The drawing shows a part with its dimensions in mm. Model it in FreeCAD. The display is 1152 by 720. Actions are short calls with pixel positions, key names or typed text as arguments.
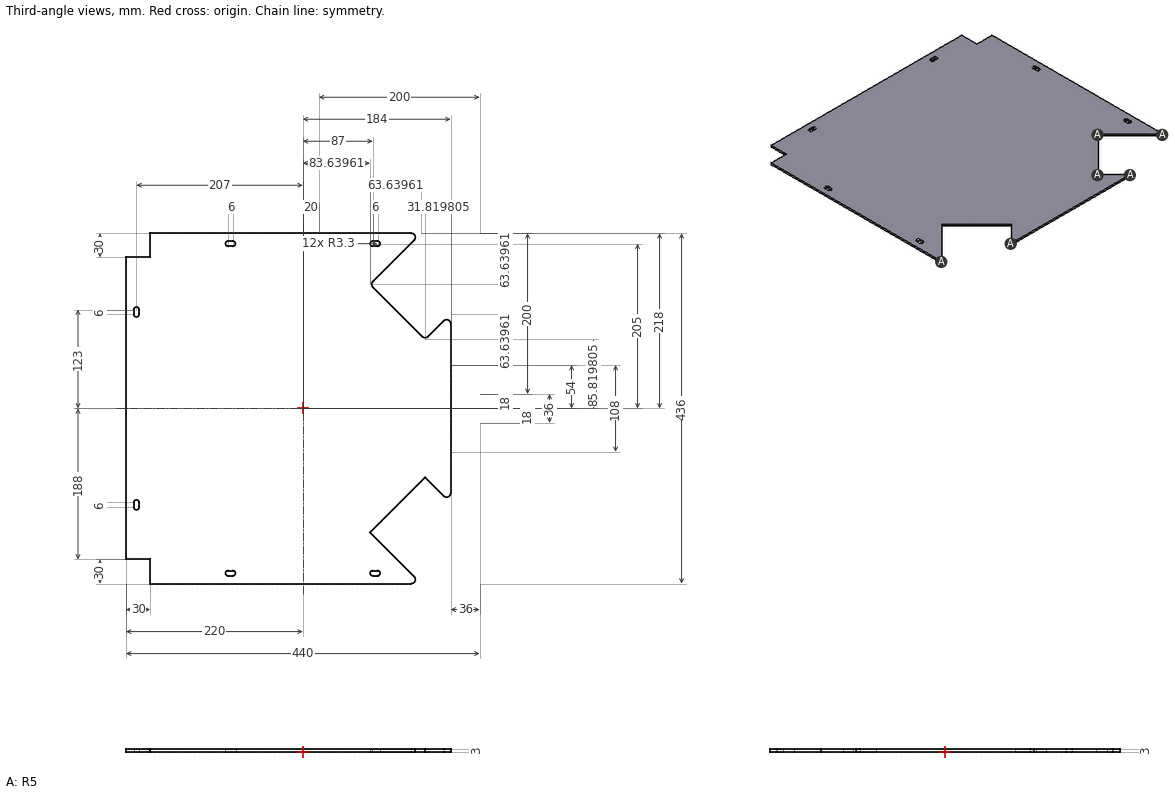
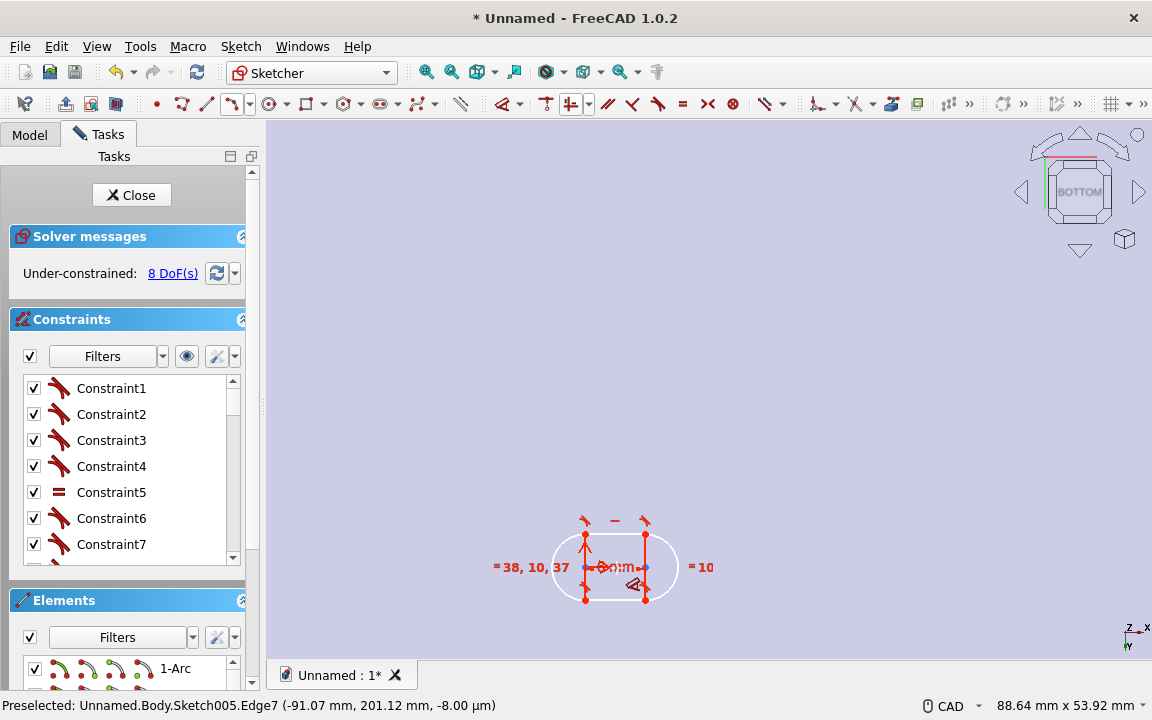
scroll(616, 539, down, 13)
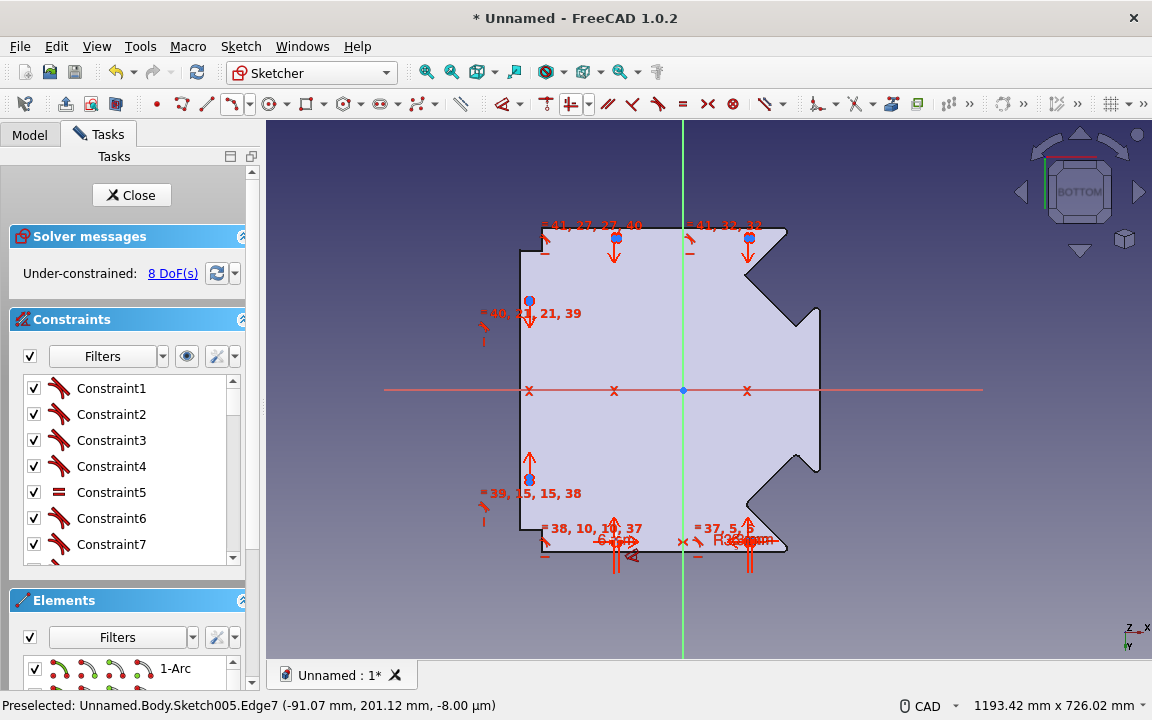
scroll(527, 481, up, 12)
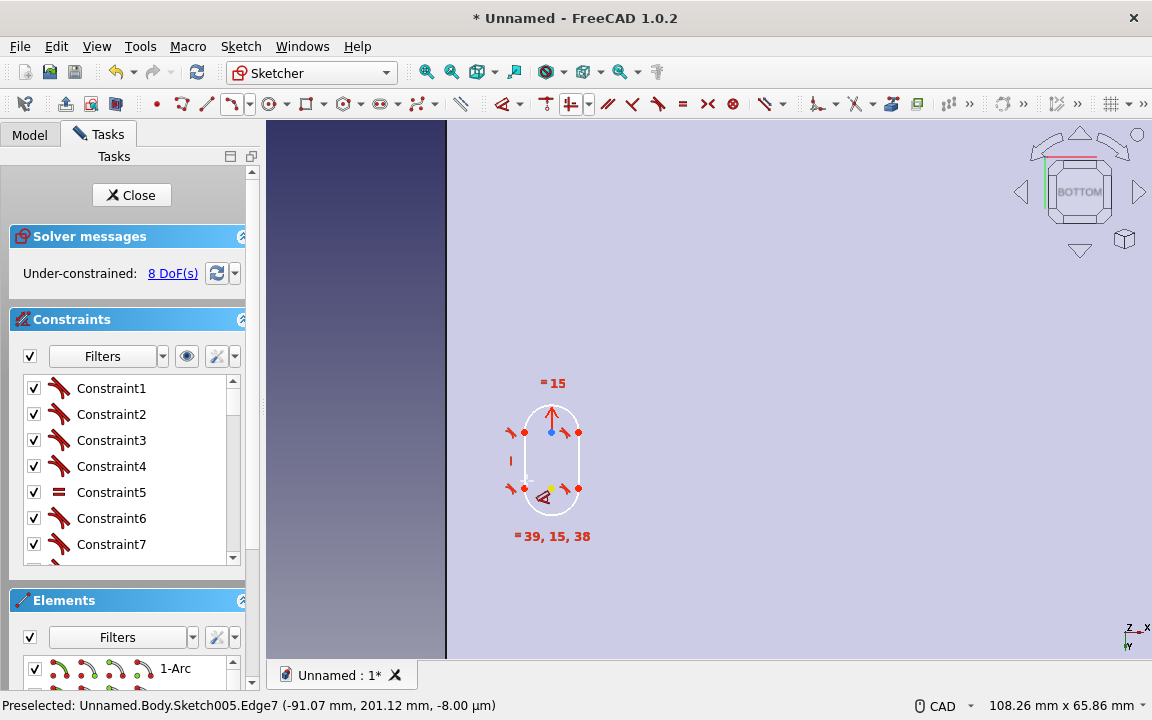
click(525, 472)
click(491, 460)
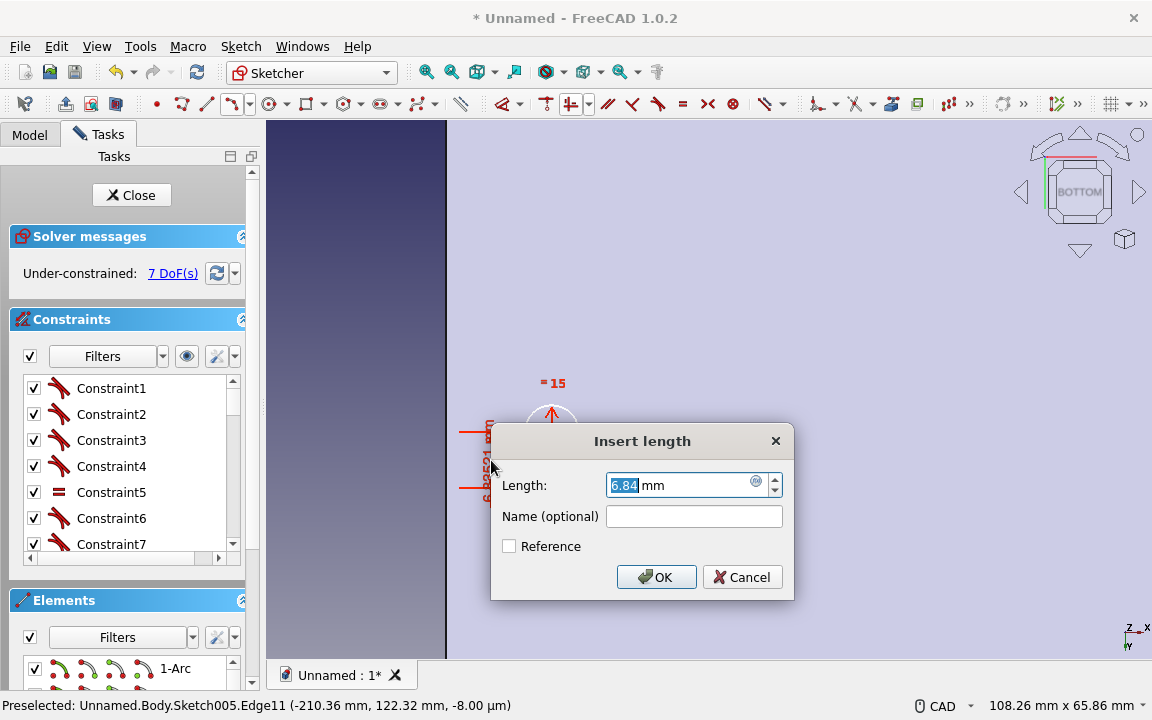
text(6)
key(Return)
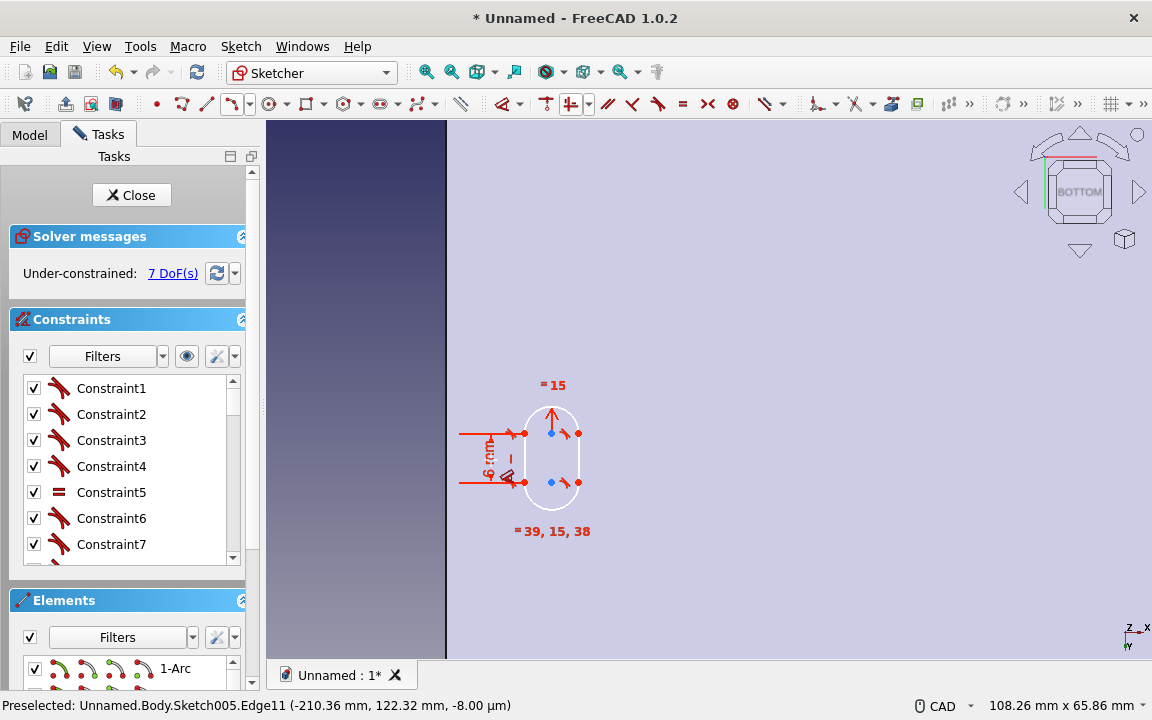
scroll(527, 481, down, 12)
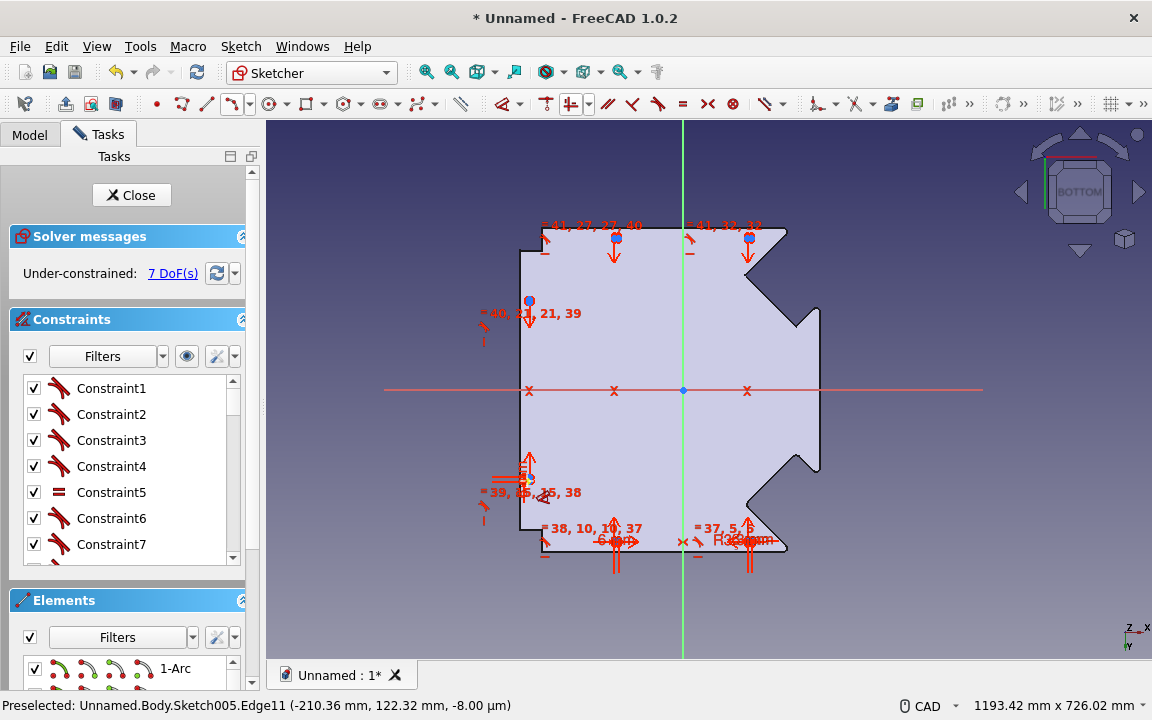
scroll(527, 302, up, 13)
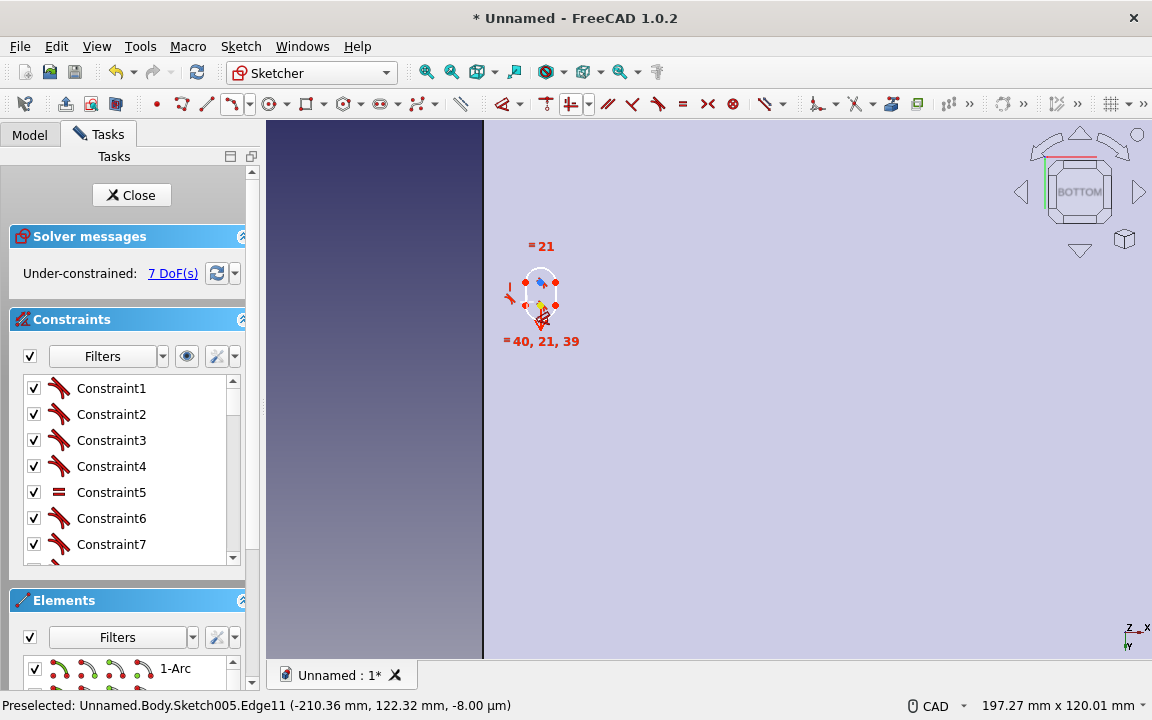
click(524, 294)
click(490, 284)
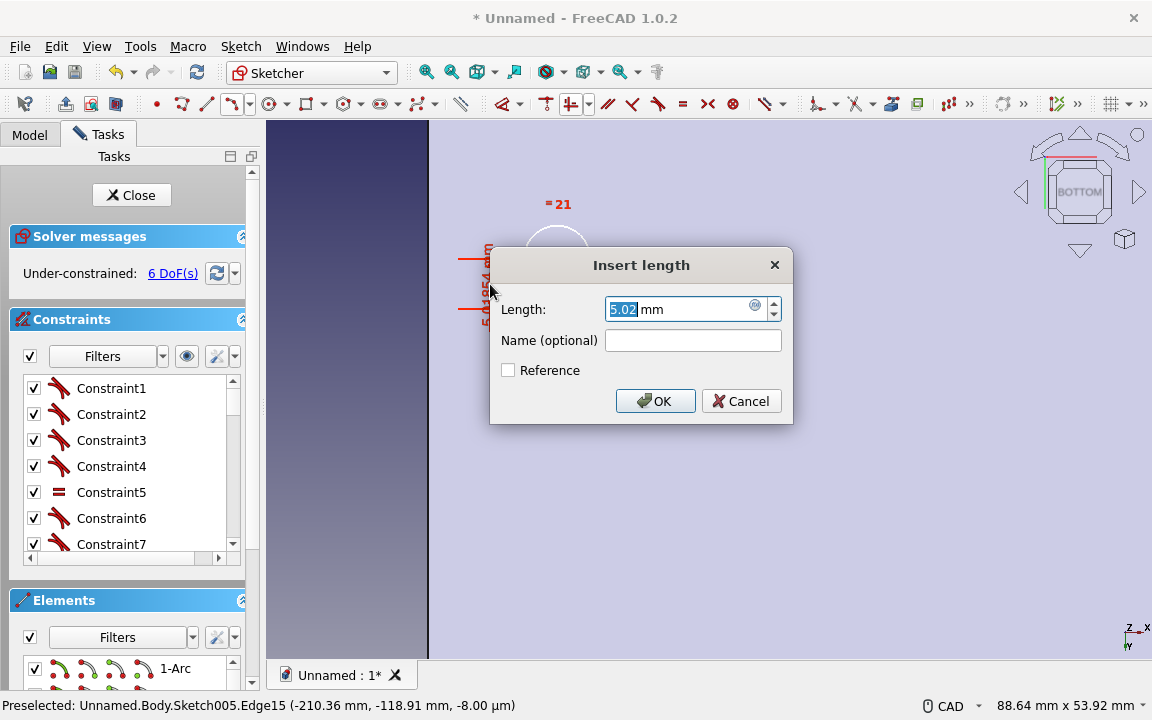
text(6)
key(Return)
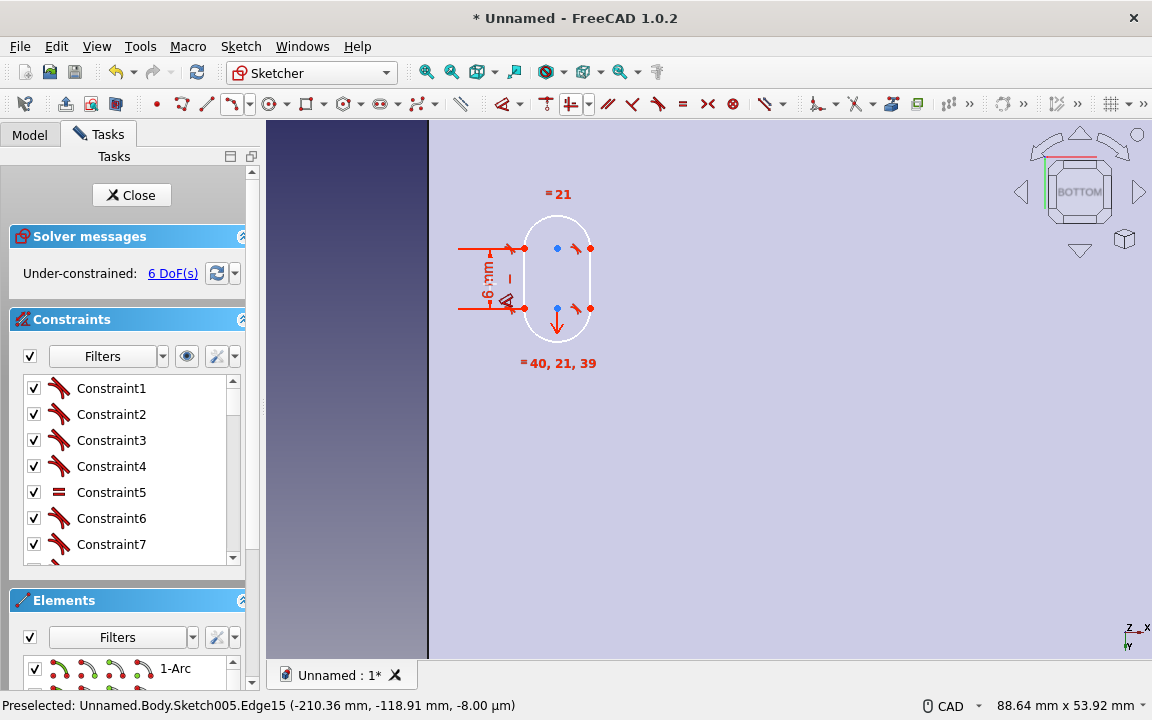
scroll(527, 302, down, 13)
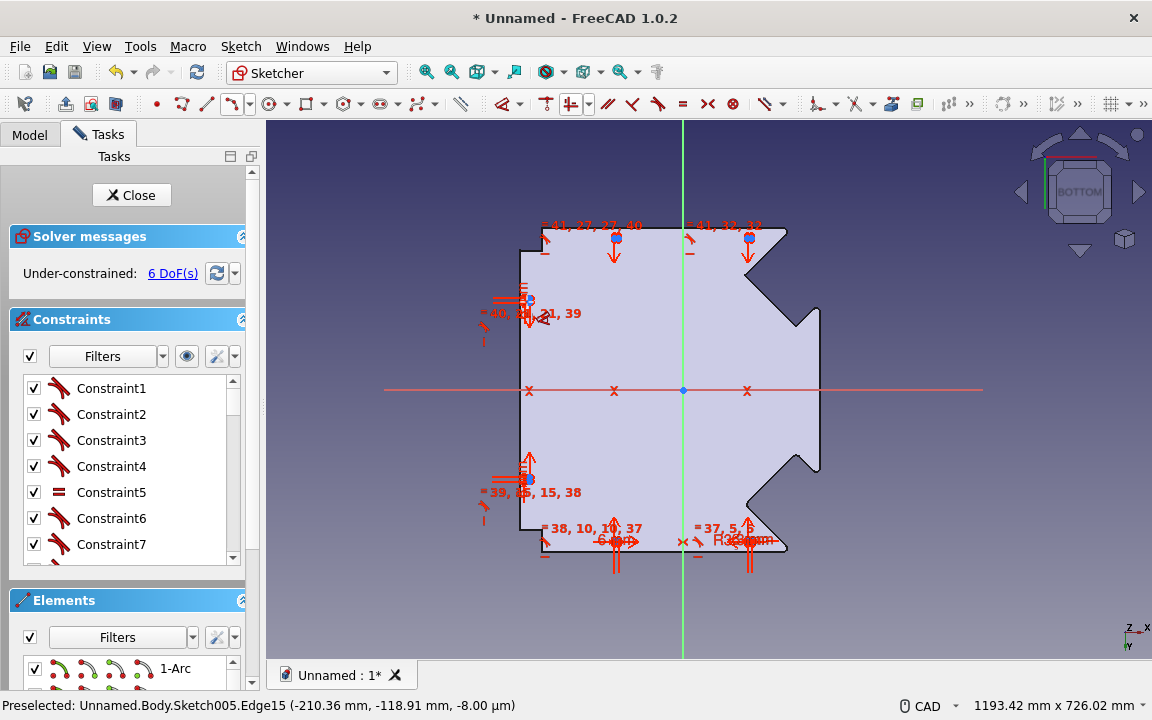
scroll(615, 236, up, 13)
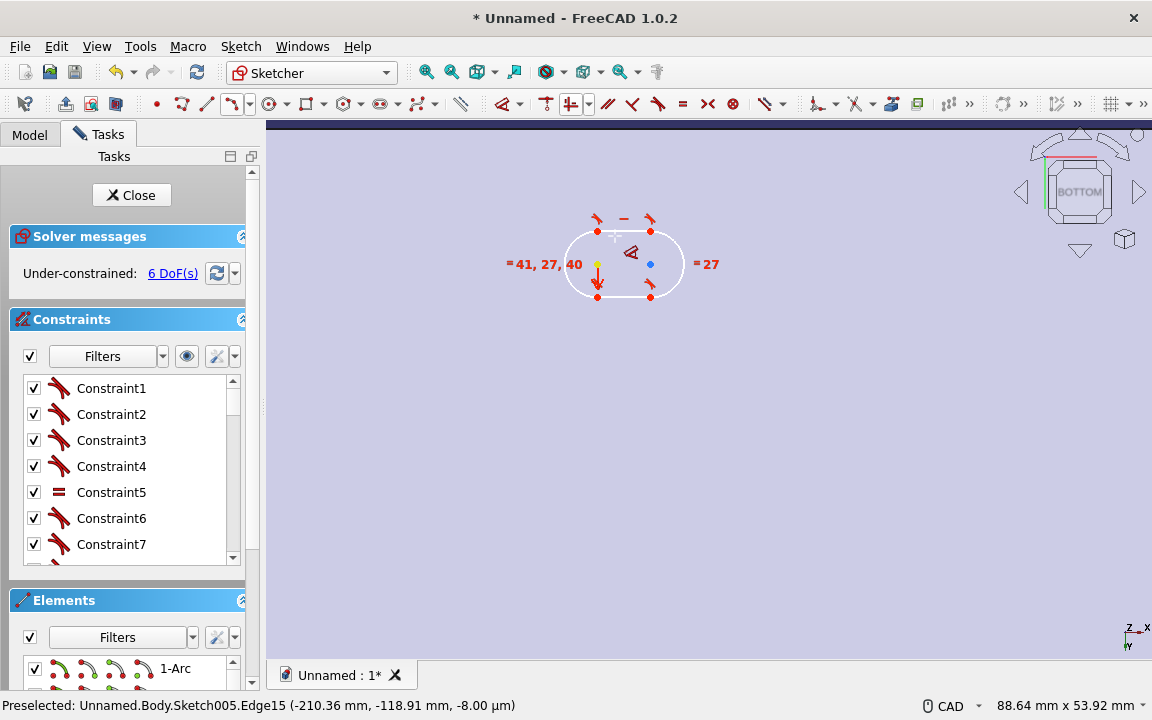
click(614, 231)
click(624, 197)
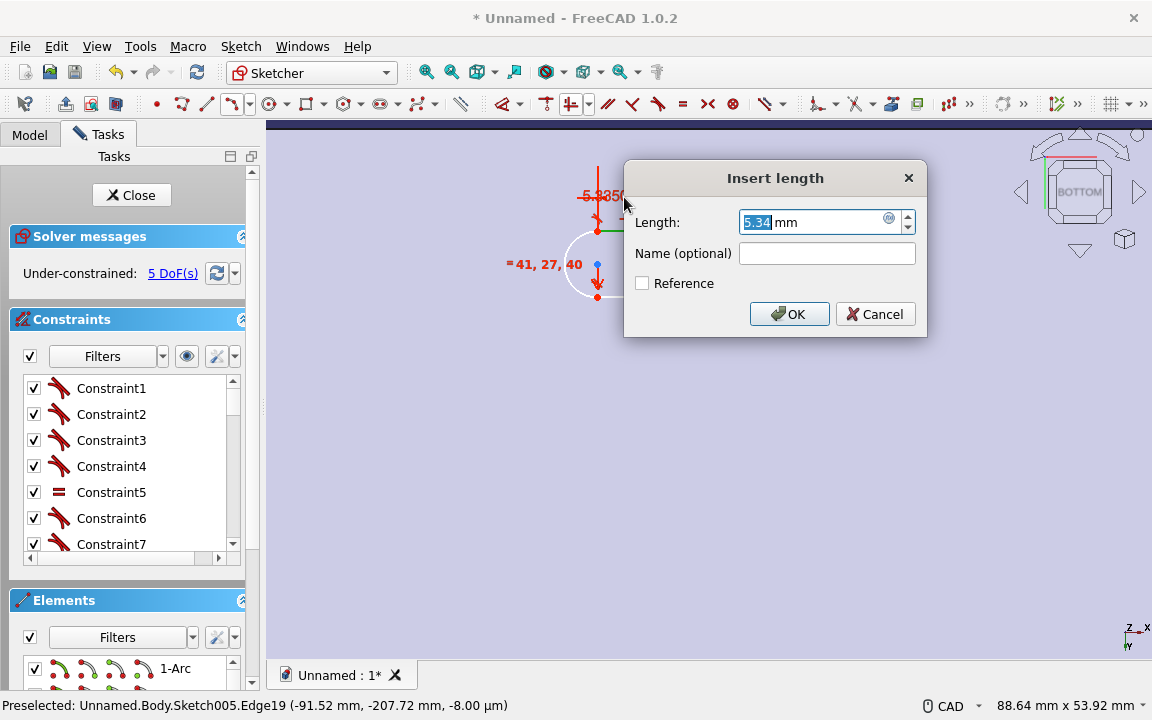
text(6)
key(Return)